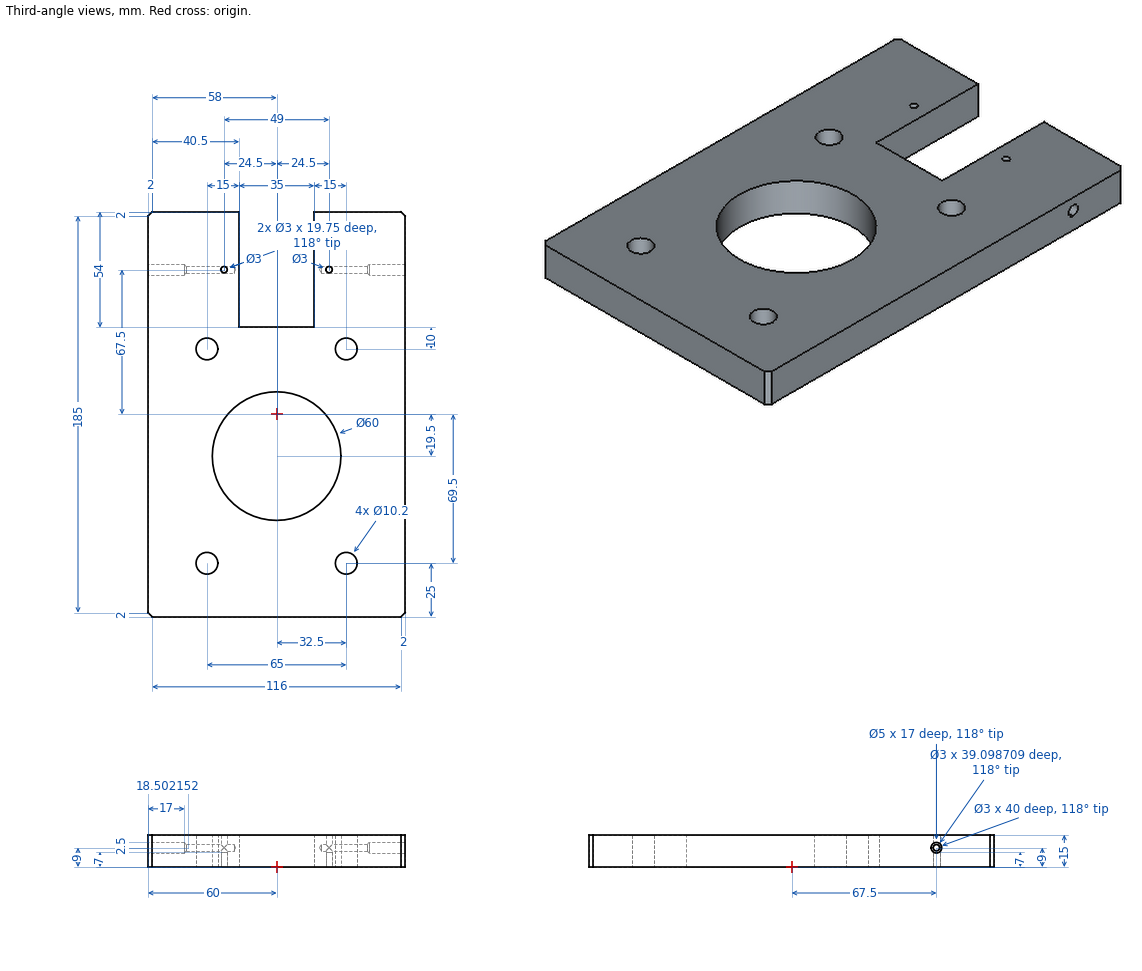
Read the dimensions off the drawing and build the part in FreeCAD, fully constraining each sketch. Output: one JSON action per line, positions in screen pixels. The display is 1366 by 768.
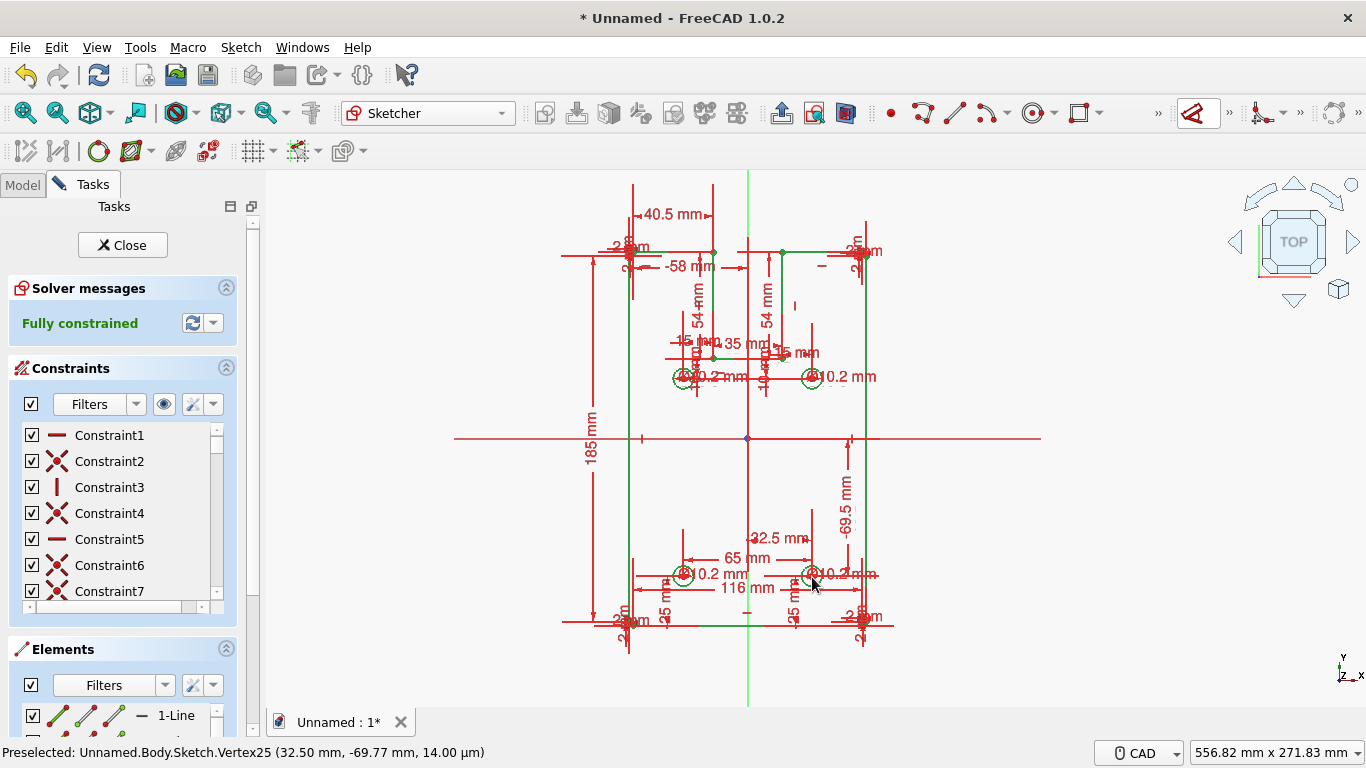
{"action": "left_click", "coordinate": [123, 245]}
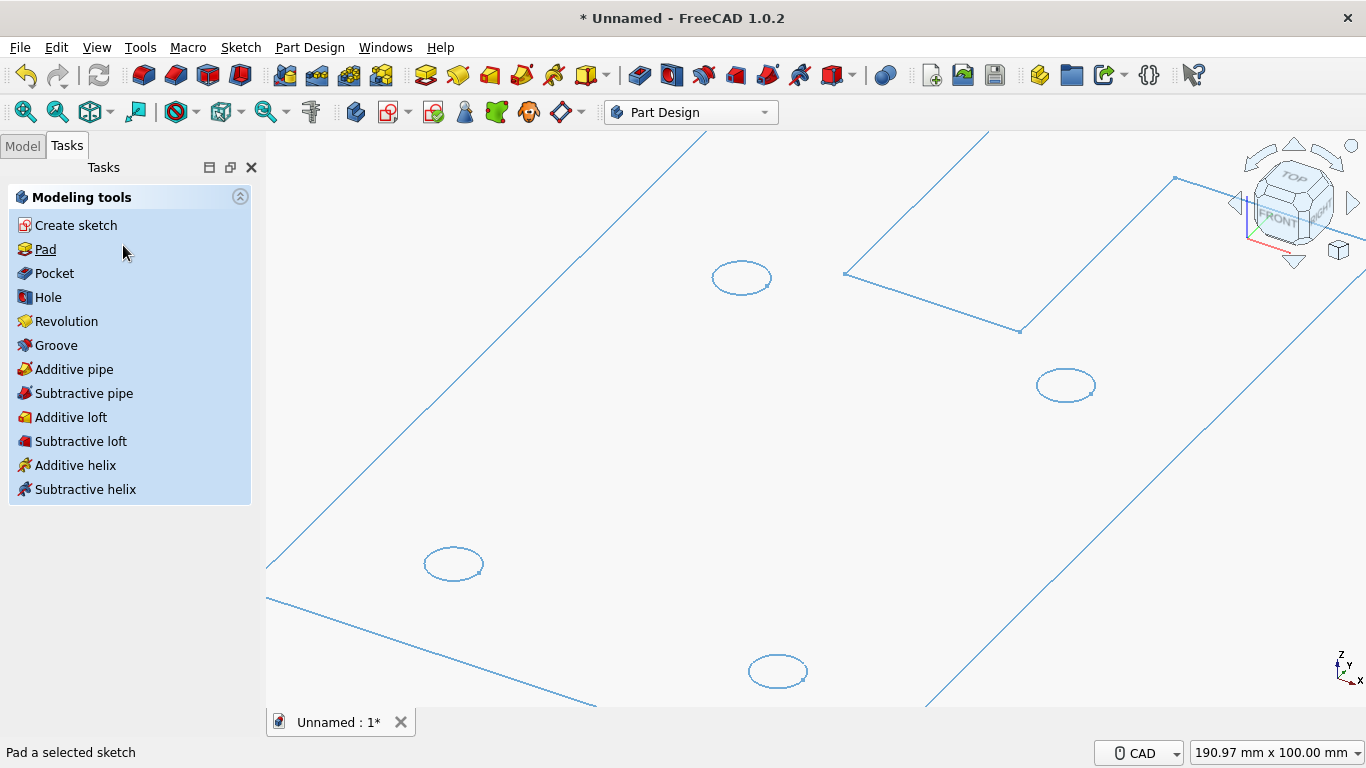
{"action": "left_click", "coordinate": [426, 76]}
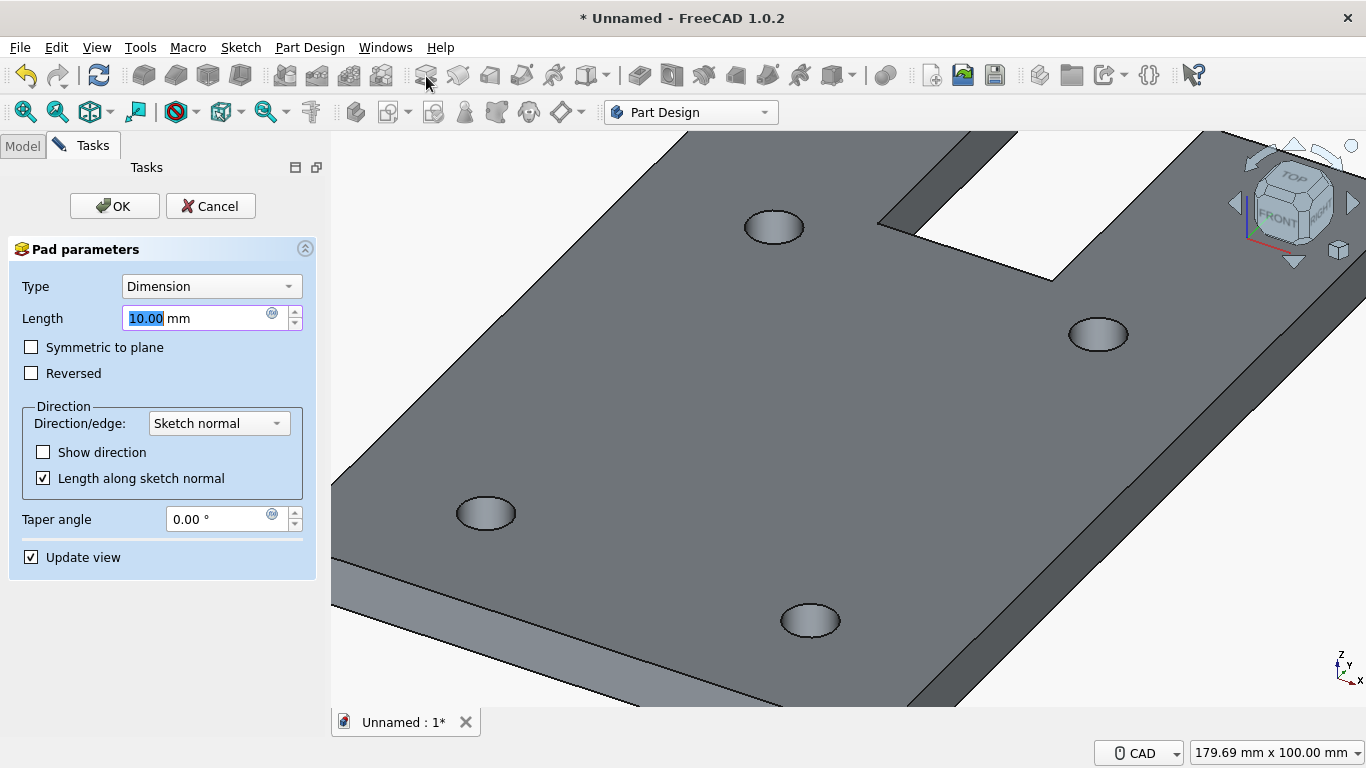
{"action": "type", "text": "15"}
{"action": "key", "text": "Tab"}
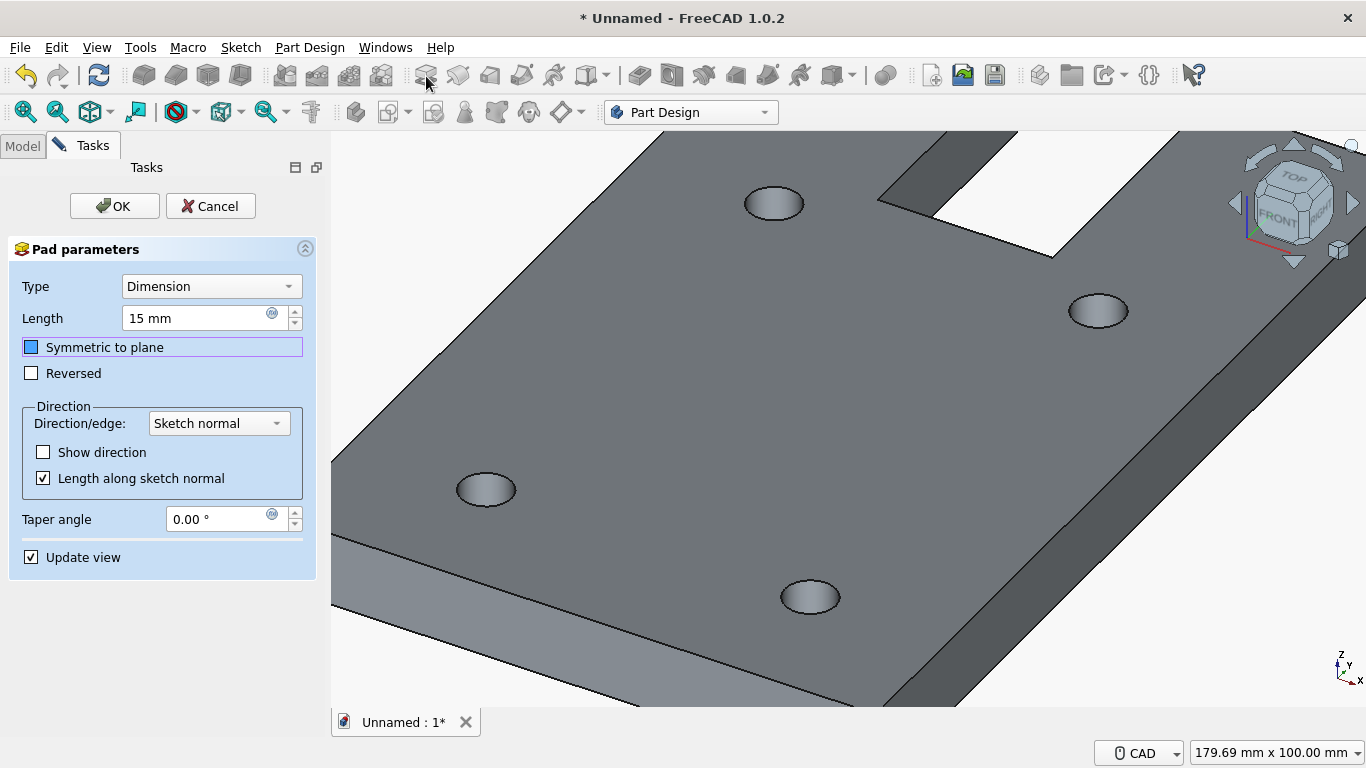
{"action": "left_click", "coordinate": [115, 206]}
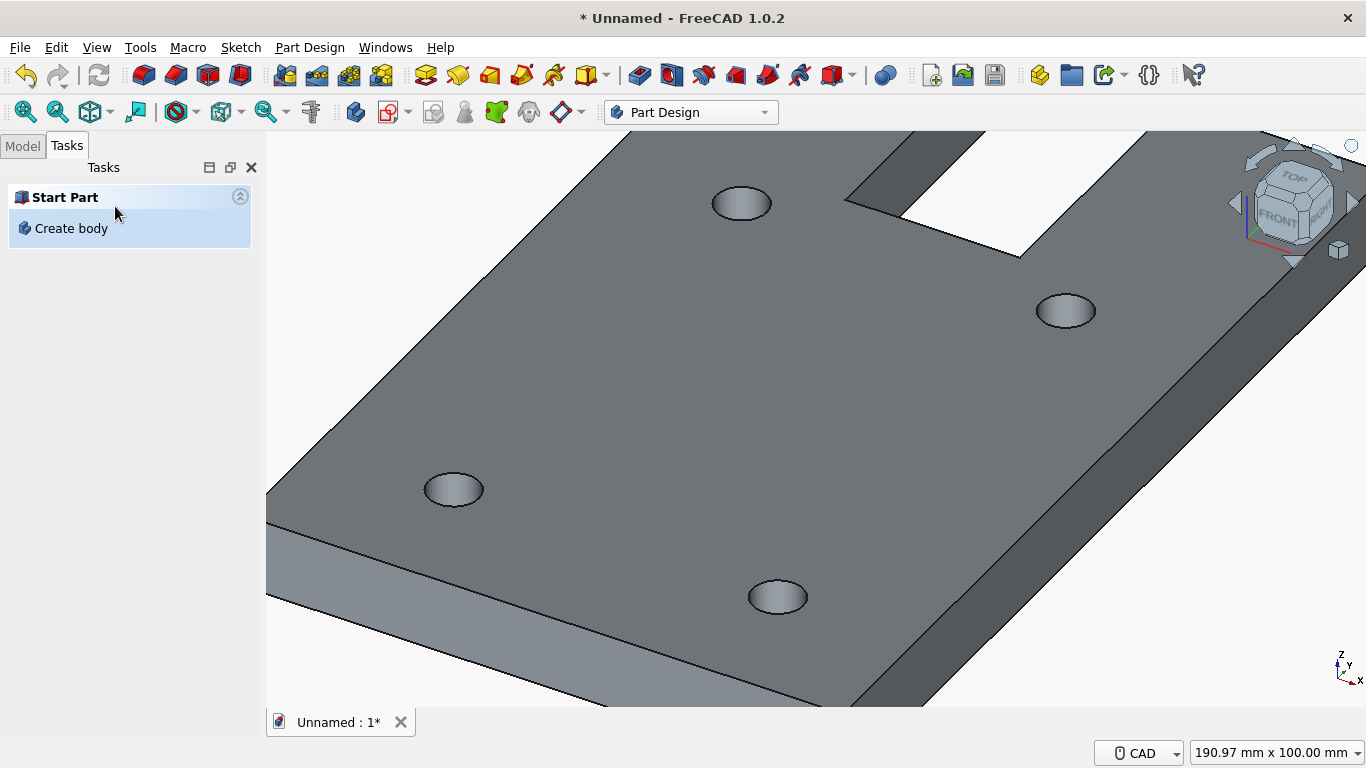
{"action": "left_click", "coordinate": [26, 112]}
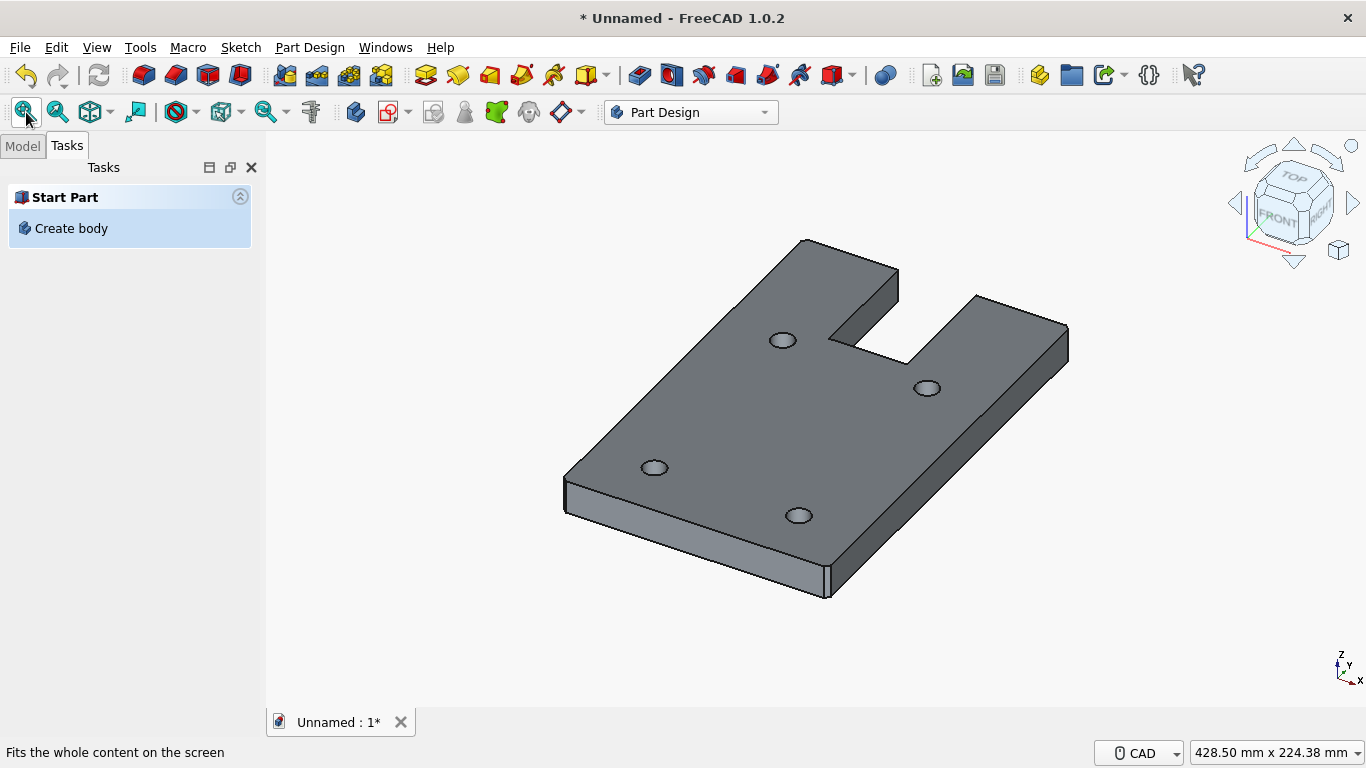
{"action": "left_click", "coordinate": [1051, 361]}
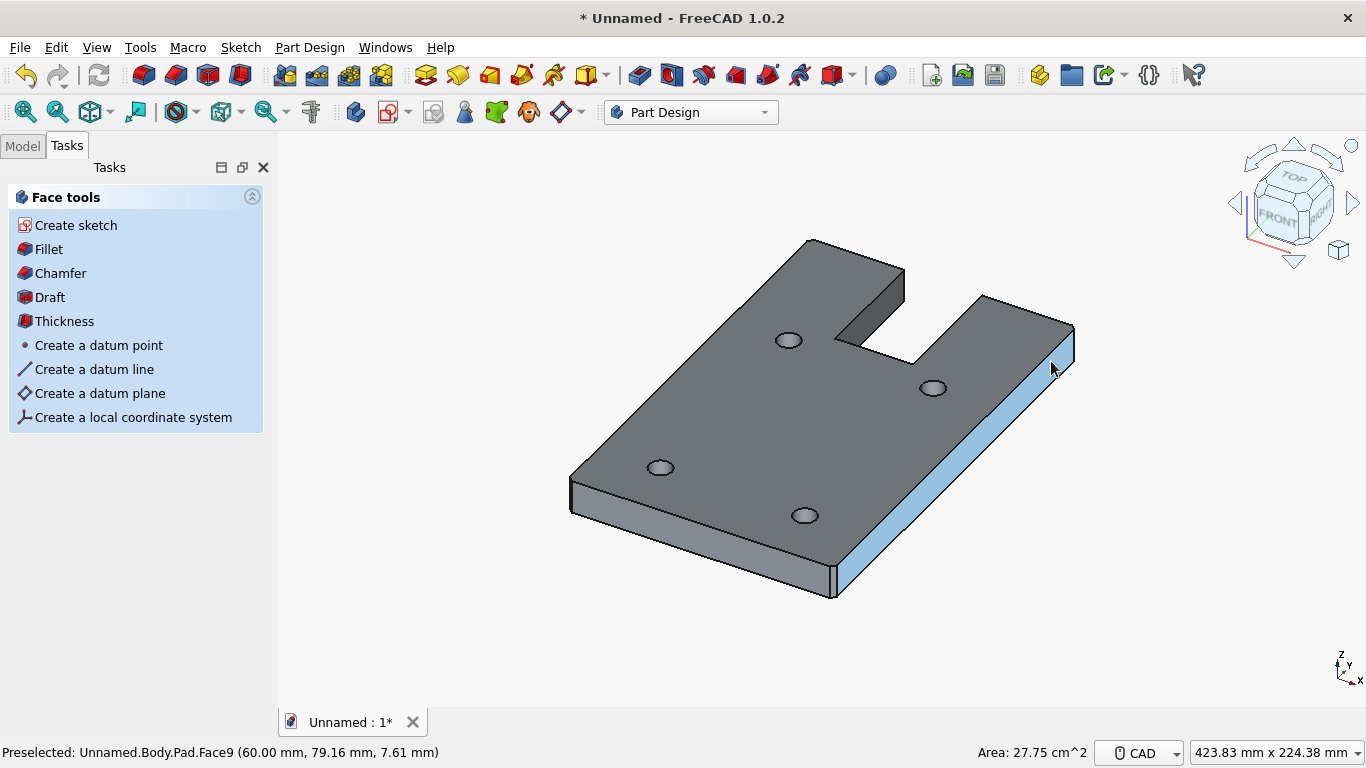
{"action": "left_click", "coordinate": [388, 112]}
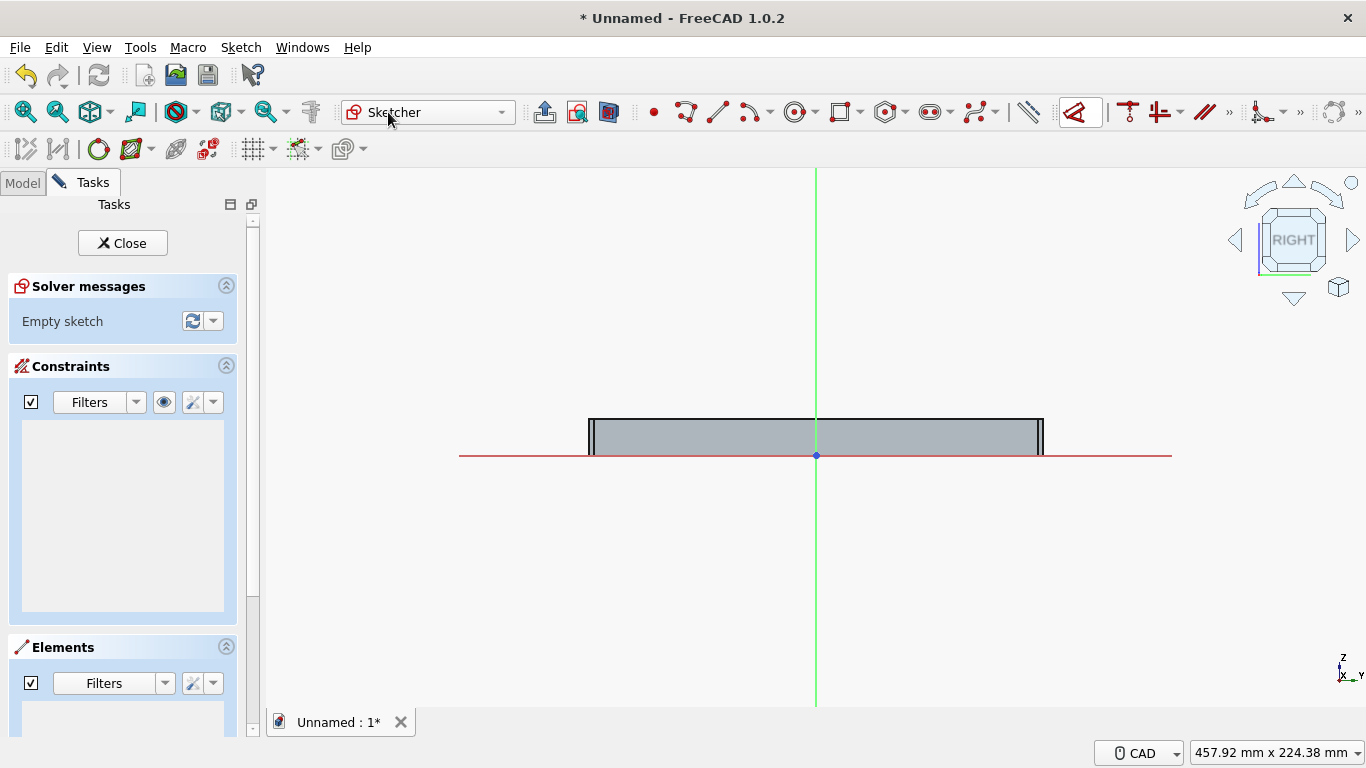
{"action": "scroll", "coordinate": [990, 434], "scroll_direction": "up", "scroll_amount": 15}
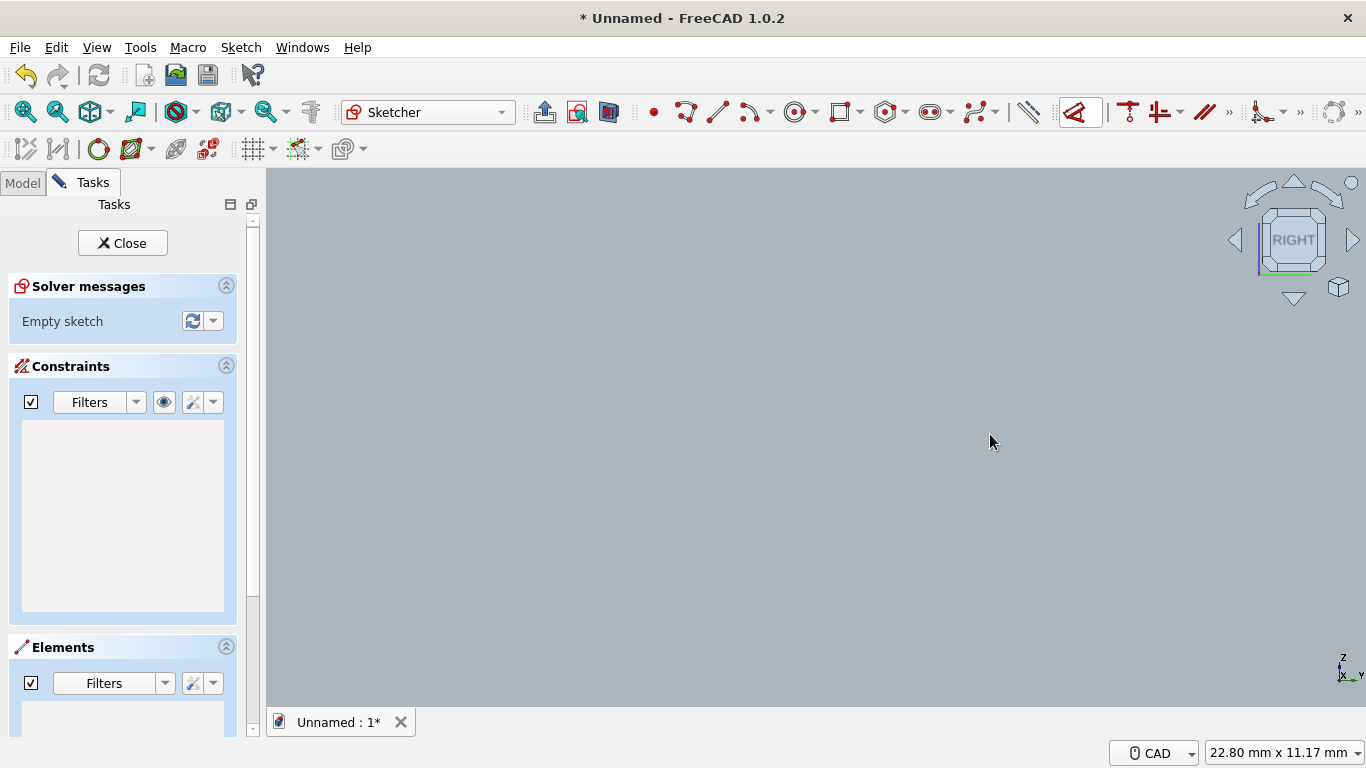
{"action": "scroll", "coordinate": [733, 410], "scroll_direction": "up", "scroll_amount": 4}